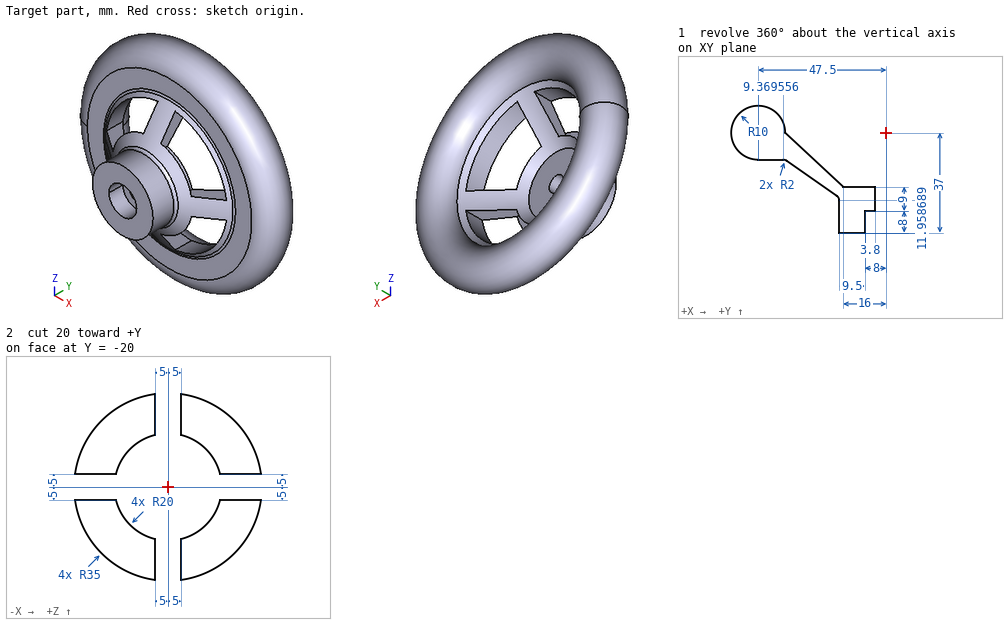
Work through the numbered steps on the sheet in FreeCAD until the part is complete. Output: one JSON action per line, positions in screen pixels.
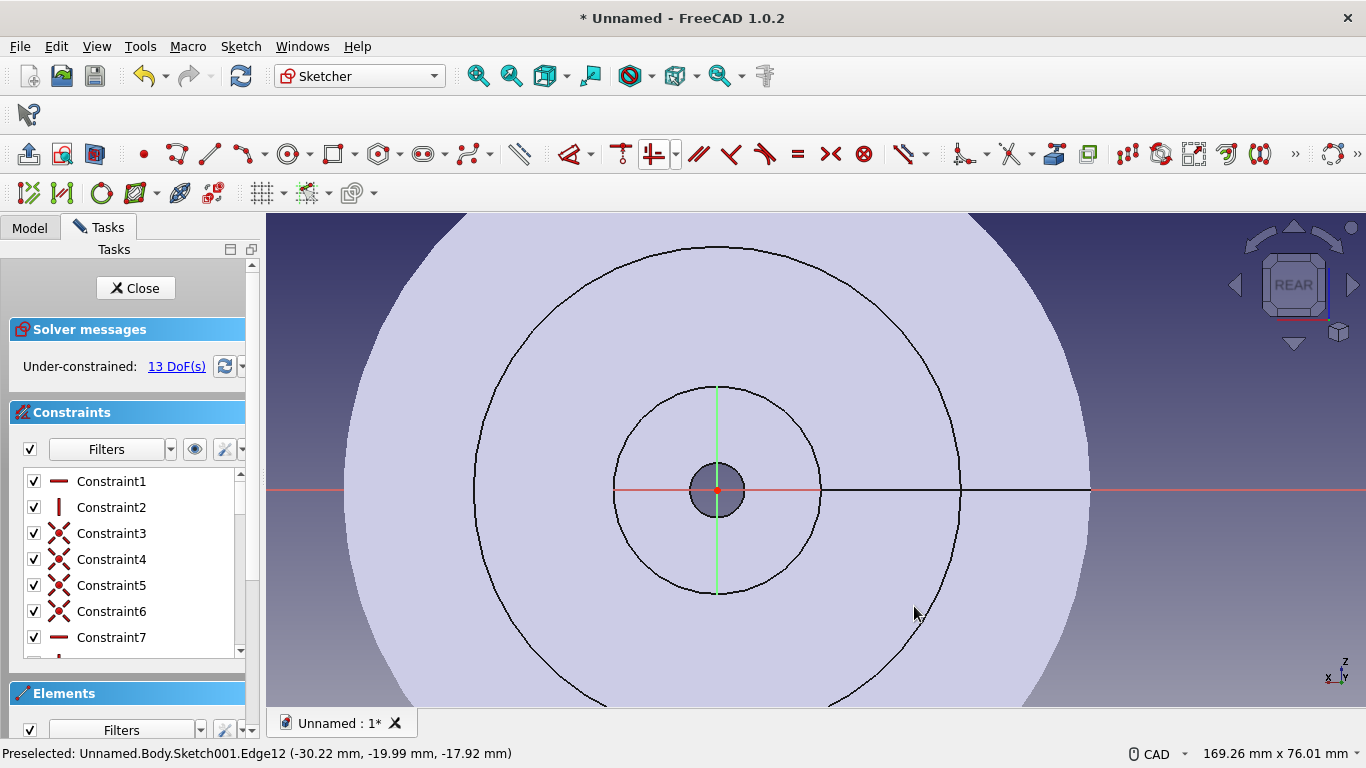
{"action": "left_click", "coordinate": [914, 377]}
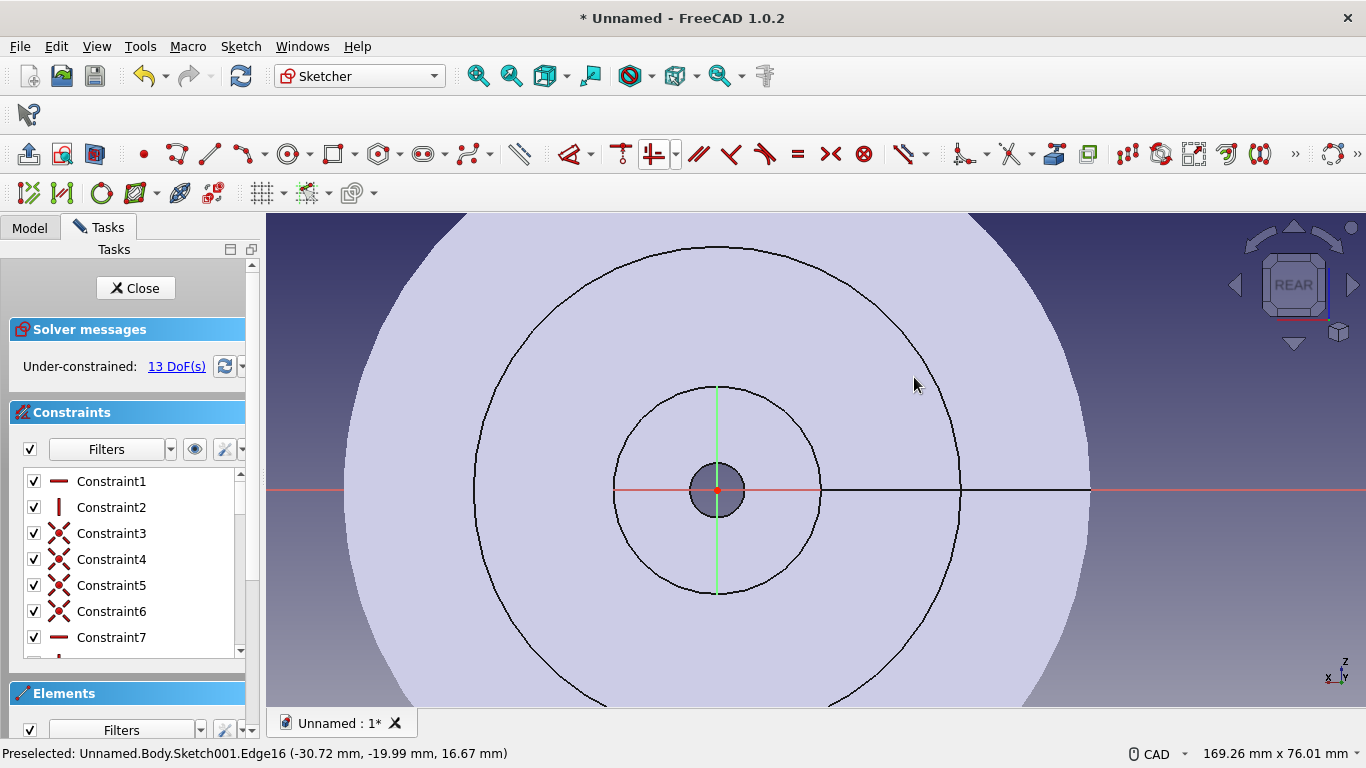
{"action": "key", "text": "e"}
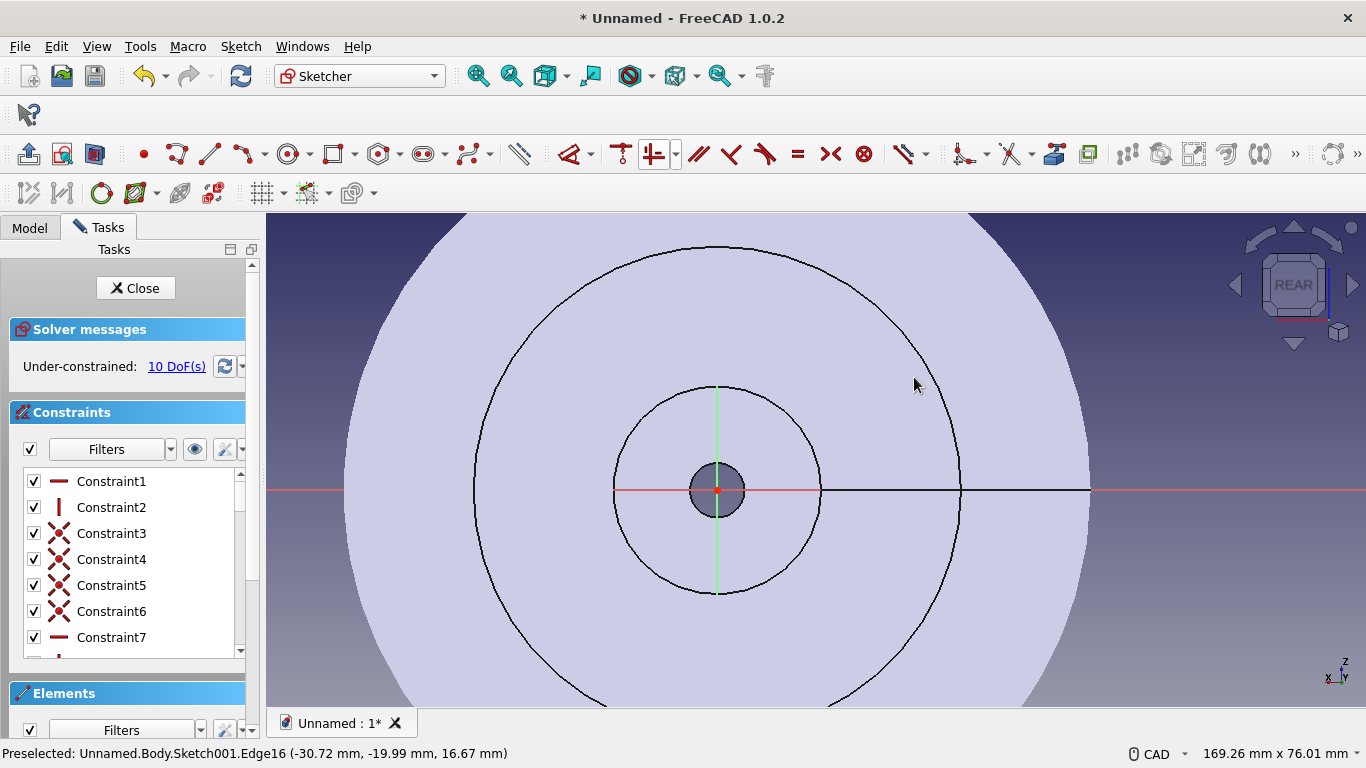
{"action": "left_click", "coordinate": [568, 154]}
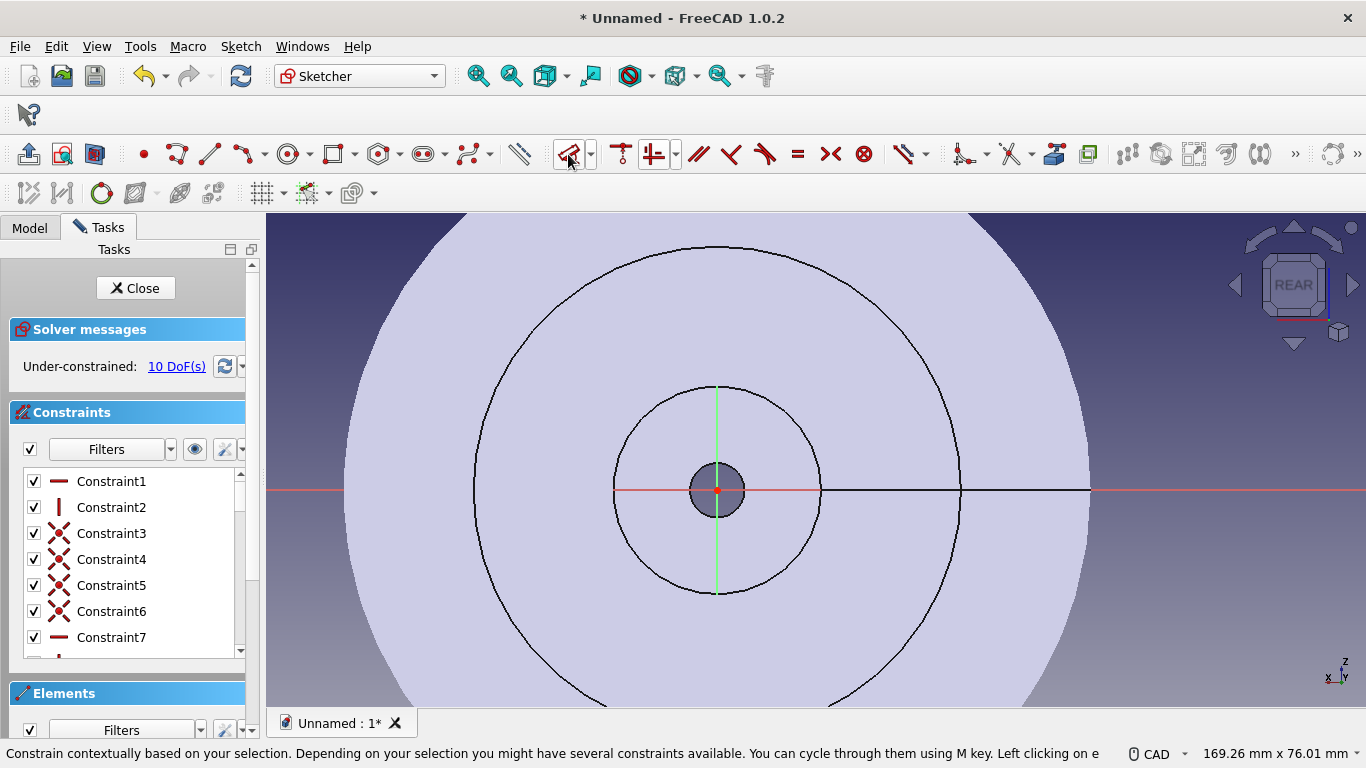
{"action": "left_click", "coordinate": [520, 606]}
{"action": "left_click", "coordinate": [492, 622]}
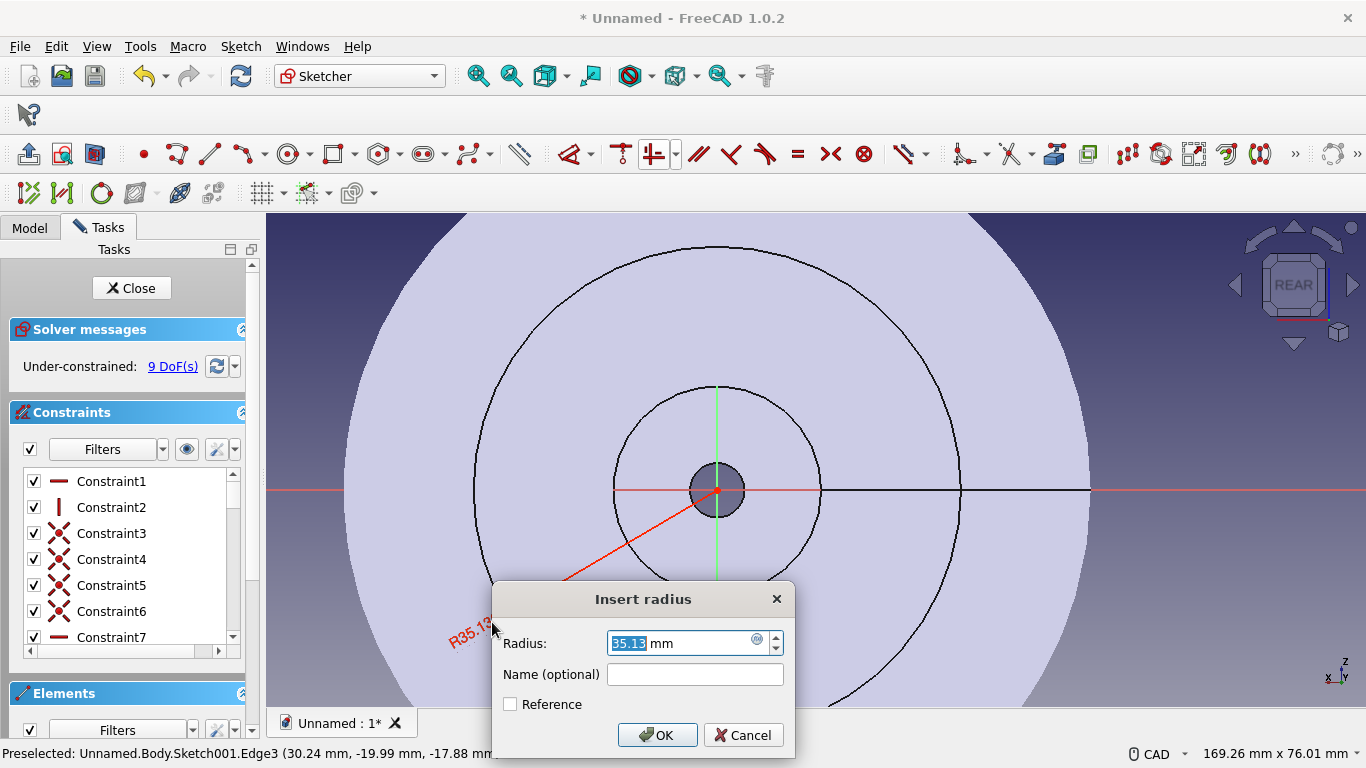
{"action": "type", "text": "35"}
{"action": "key", "text": "Return"}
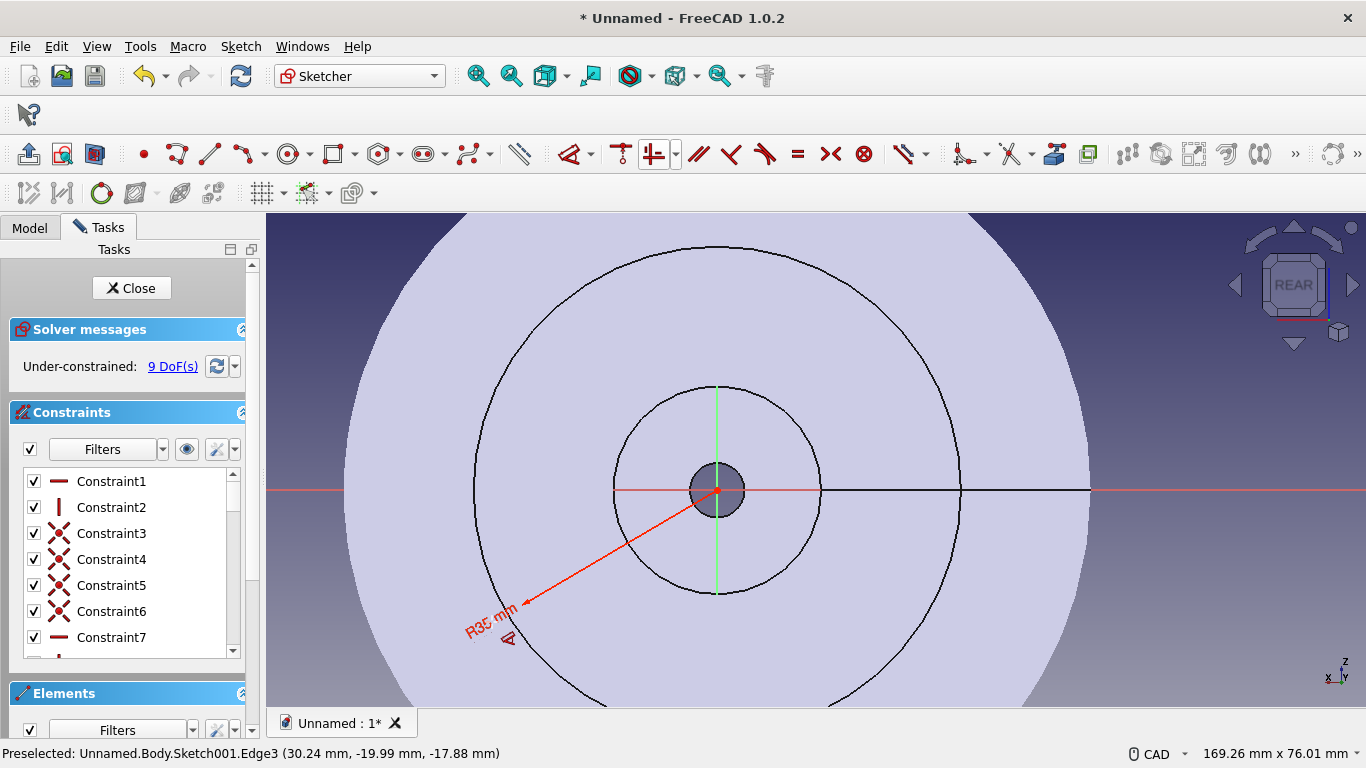
{"action": "left_click", "coordinate": [608, 562]}
{"action": "left_click", "coordinate": [581, 580]}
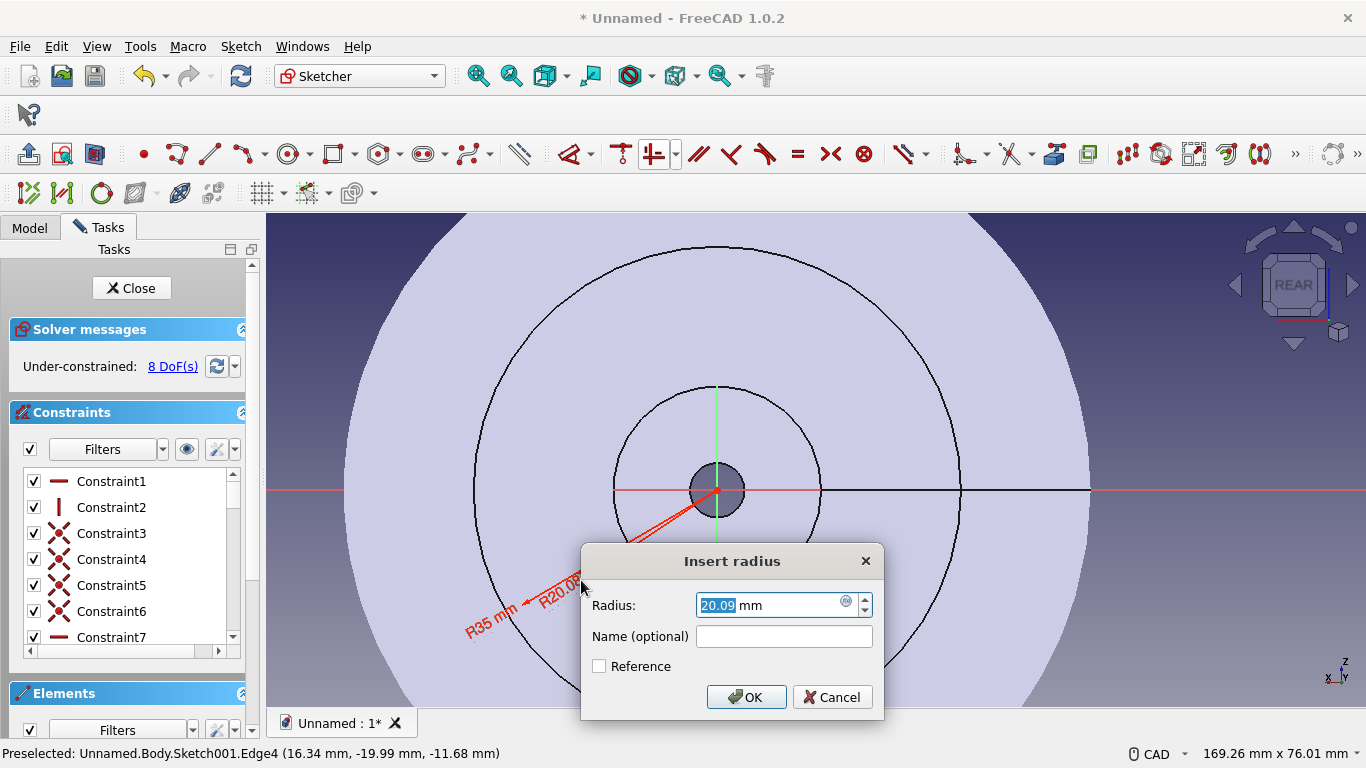
{"action": "type", "text": "20"}
{"action": "key", "text": "Return"}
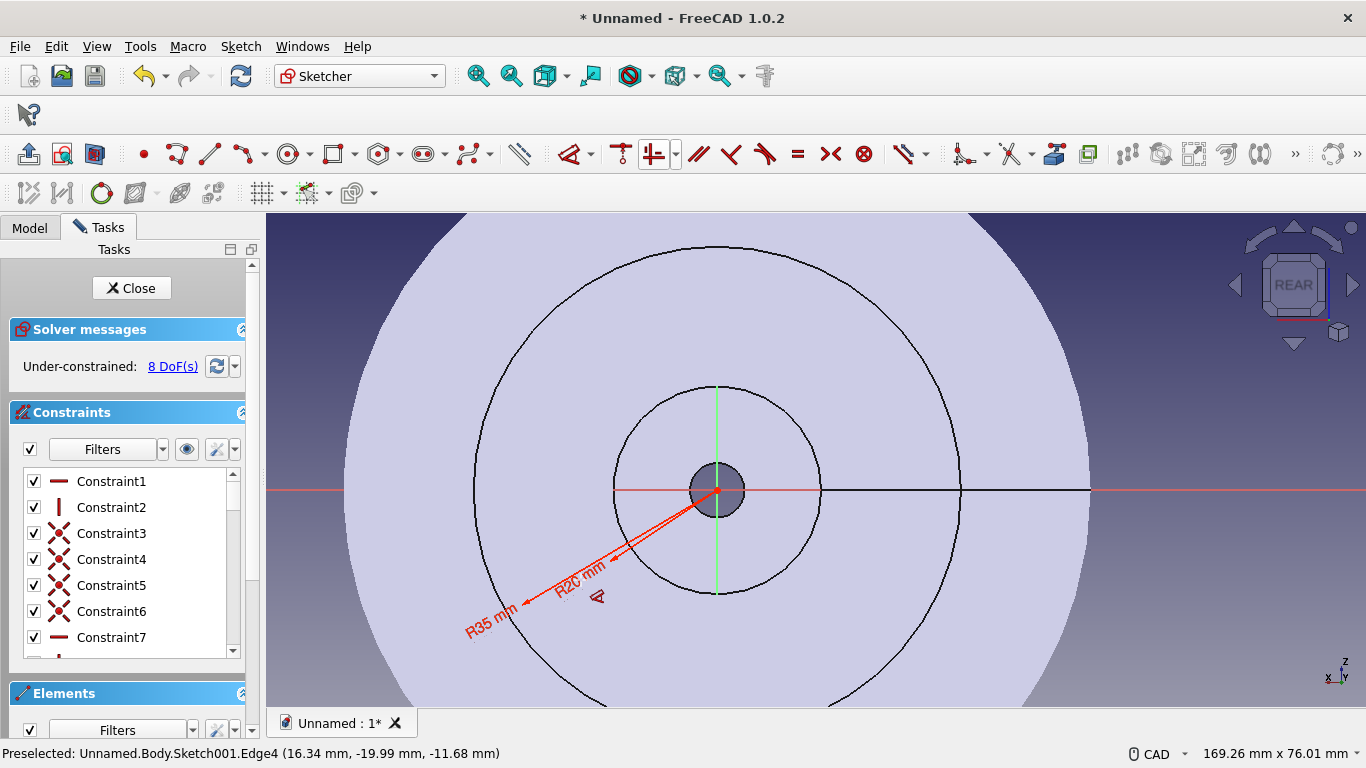
{"action": "scroll", "coordinate": [592, 524], "scroll_direction": "up", "scroll_amount": 2}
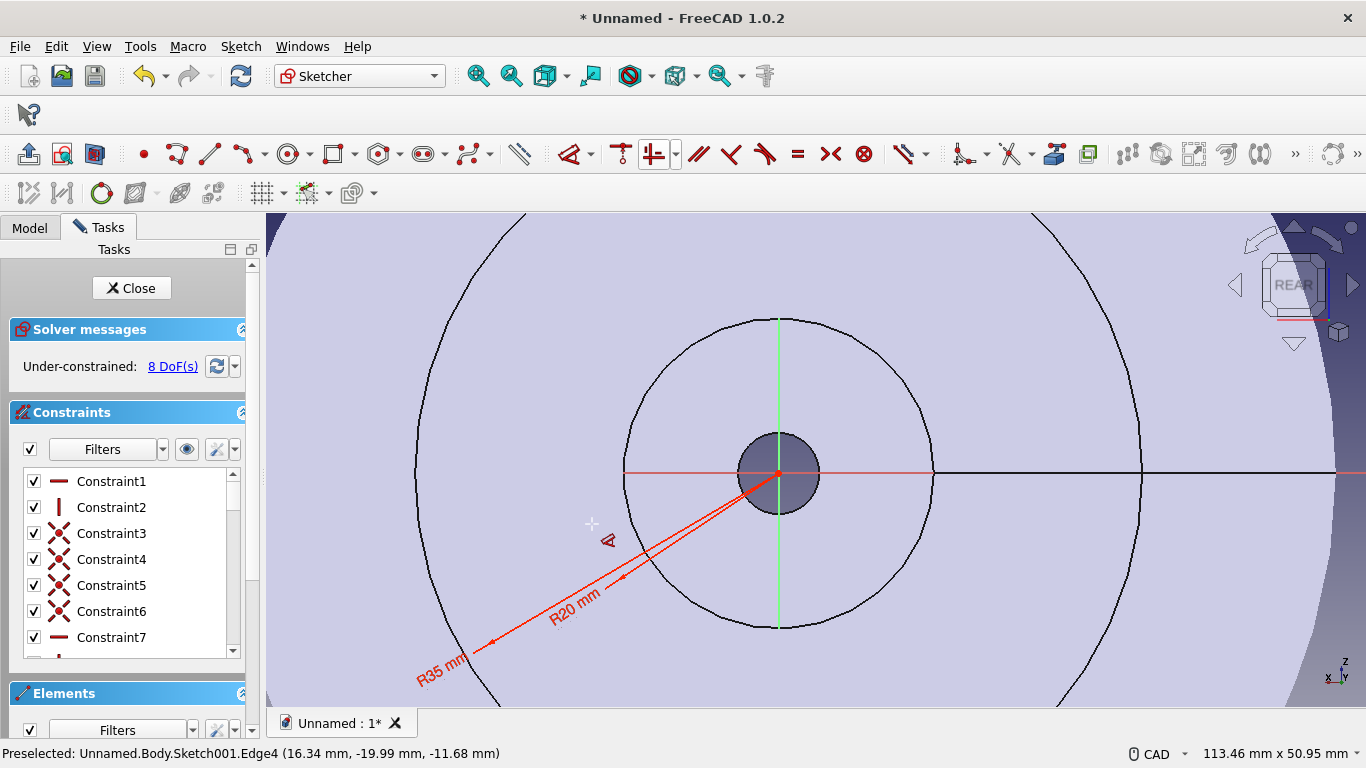
{"action": "left_click", "coordinate": [591, 523]}
{"action": "left_click", "coordinate": [557, 498]}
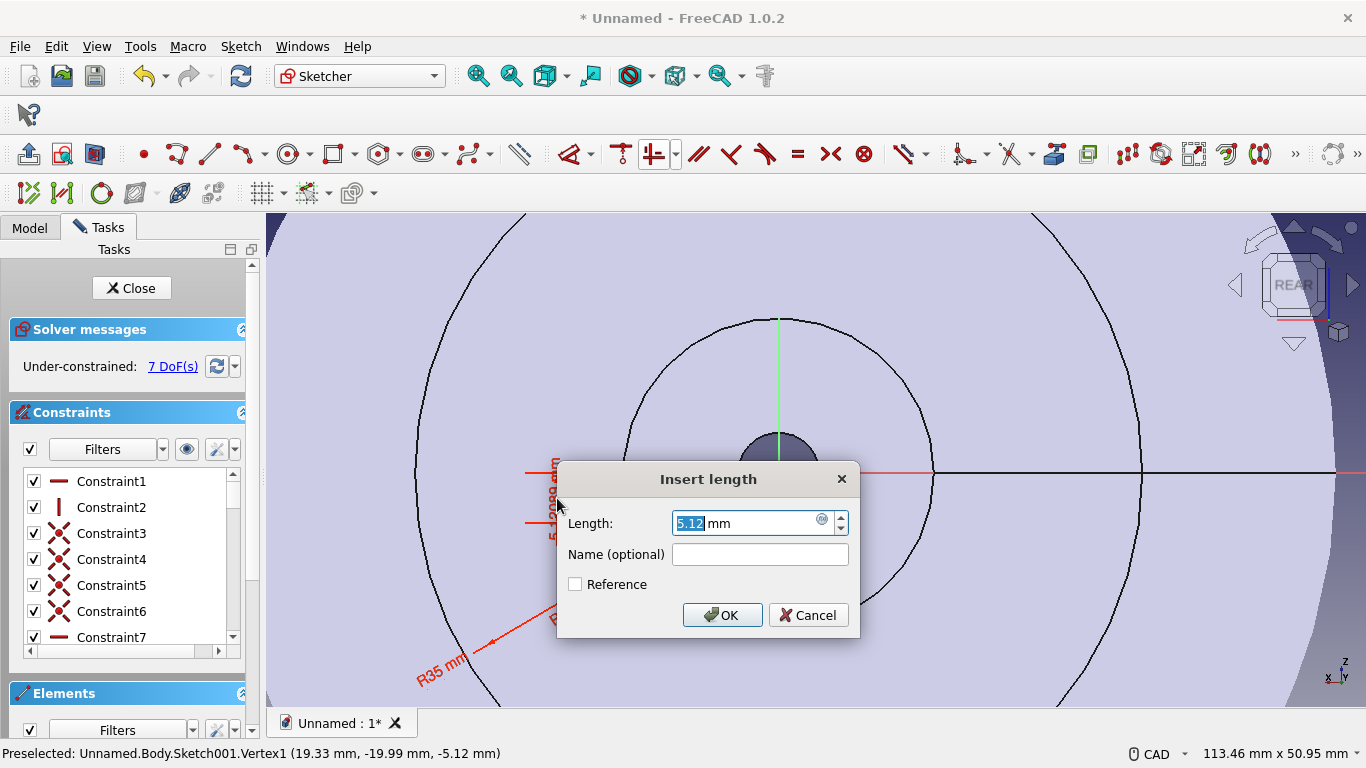
{"action": "type", "text": "5"}
{"action": "key", "text": "Return"}